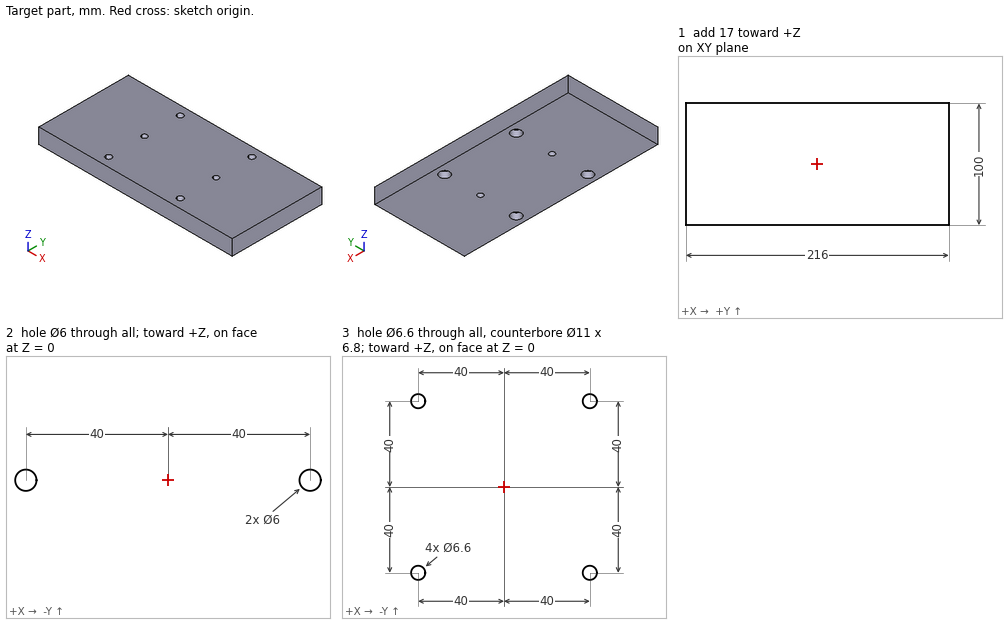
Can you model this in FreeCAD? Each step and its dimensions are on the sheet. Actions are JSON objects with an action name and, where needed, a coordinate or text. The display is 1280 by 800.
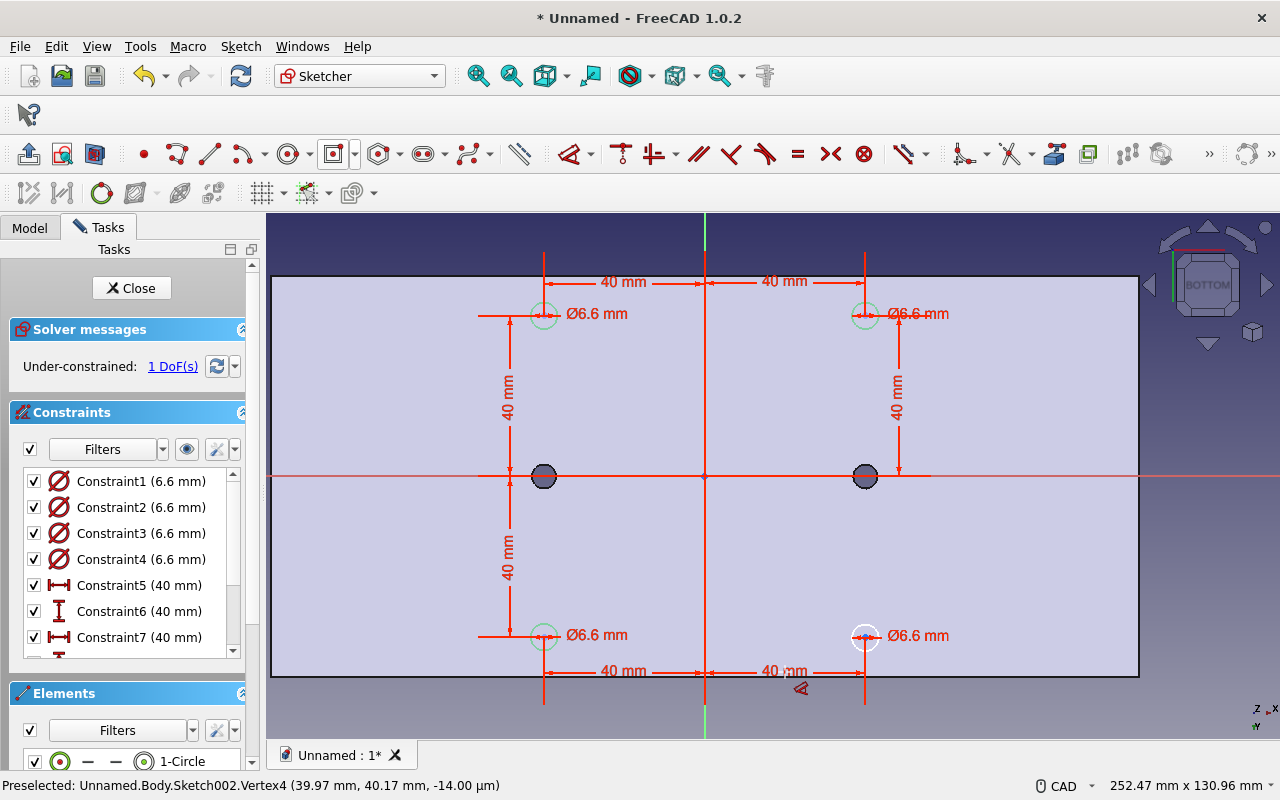
{"action": "left_click", "coordinate": [865, 638]}
{"action": "left_click", "coordinate": [899, 557]}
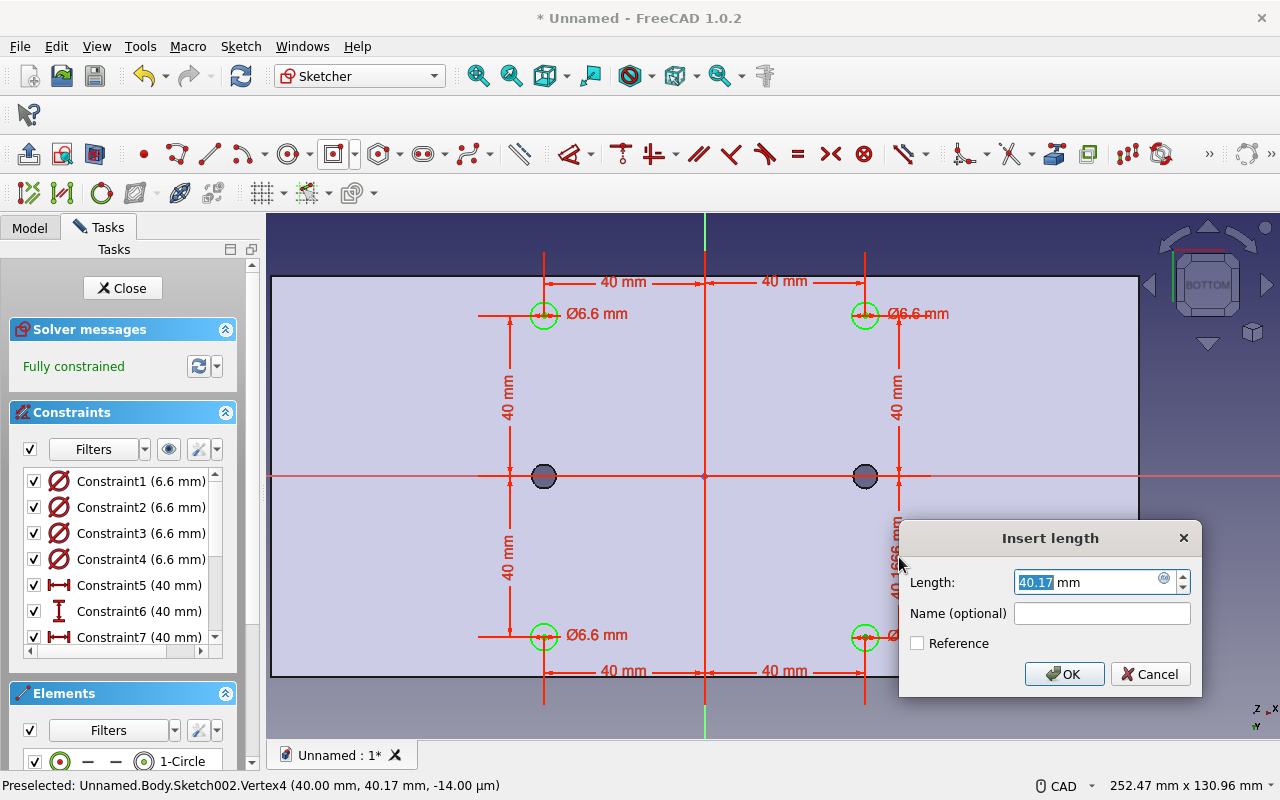
{"action": "type", "text": "40"}
{"action": "key", "text": "Return"}
{"action": "key", "text": "Escape"}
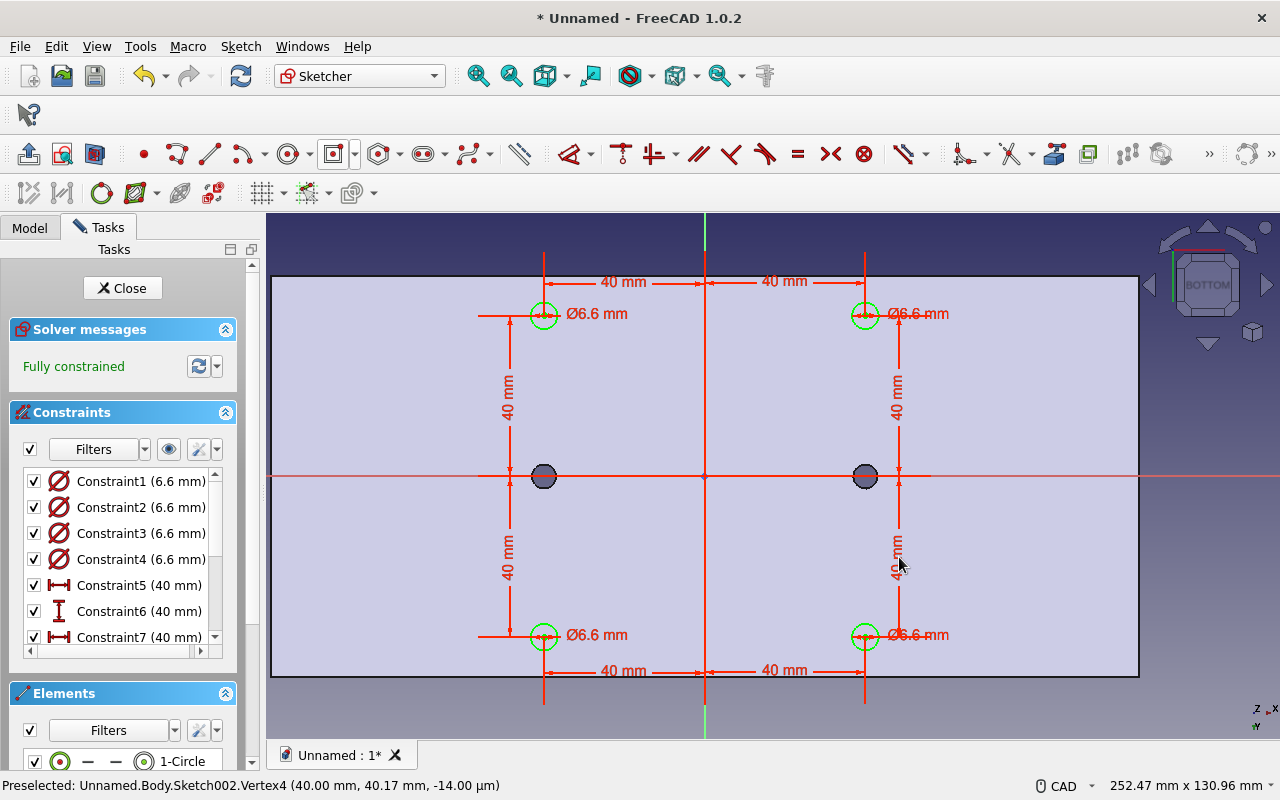
{"action": "left_click", "coordinate": [123, 288]}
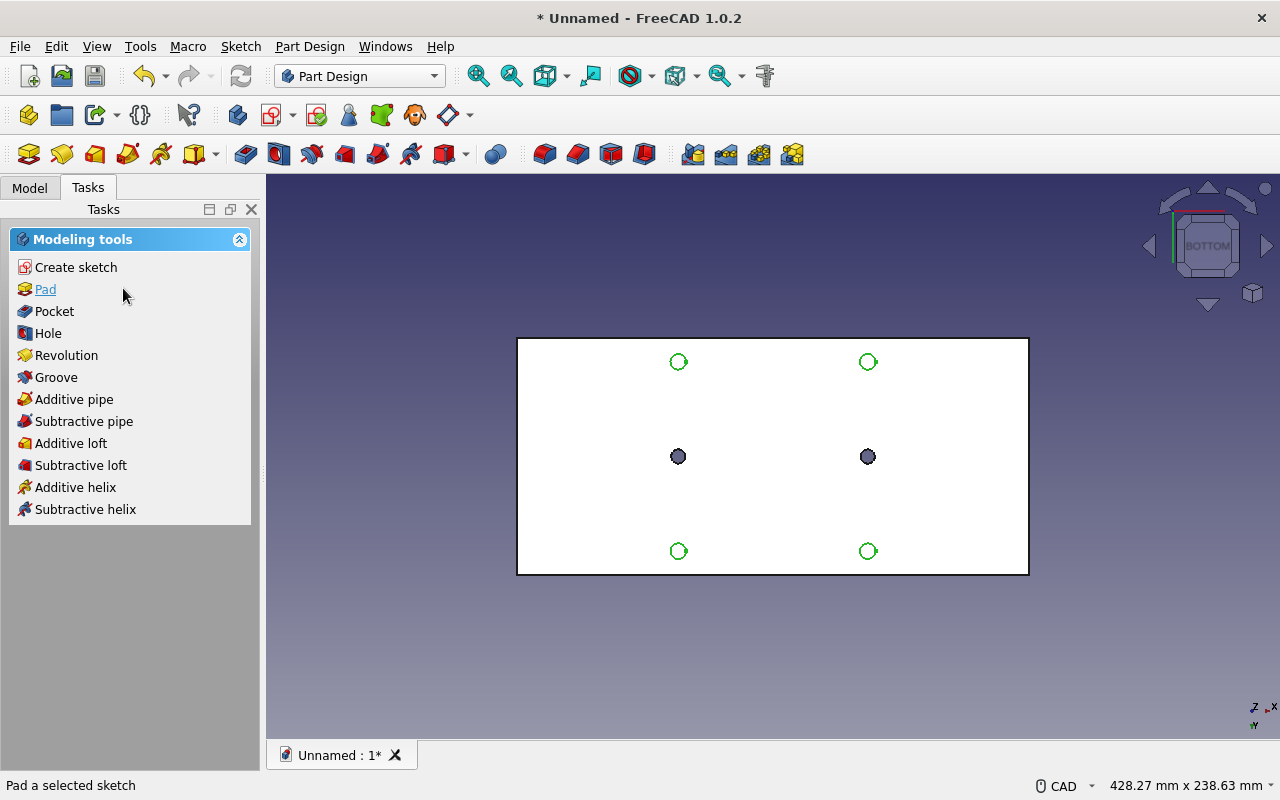
{"action": "left_click", "coordinate": [279, 154]}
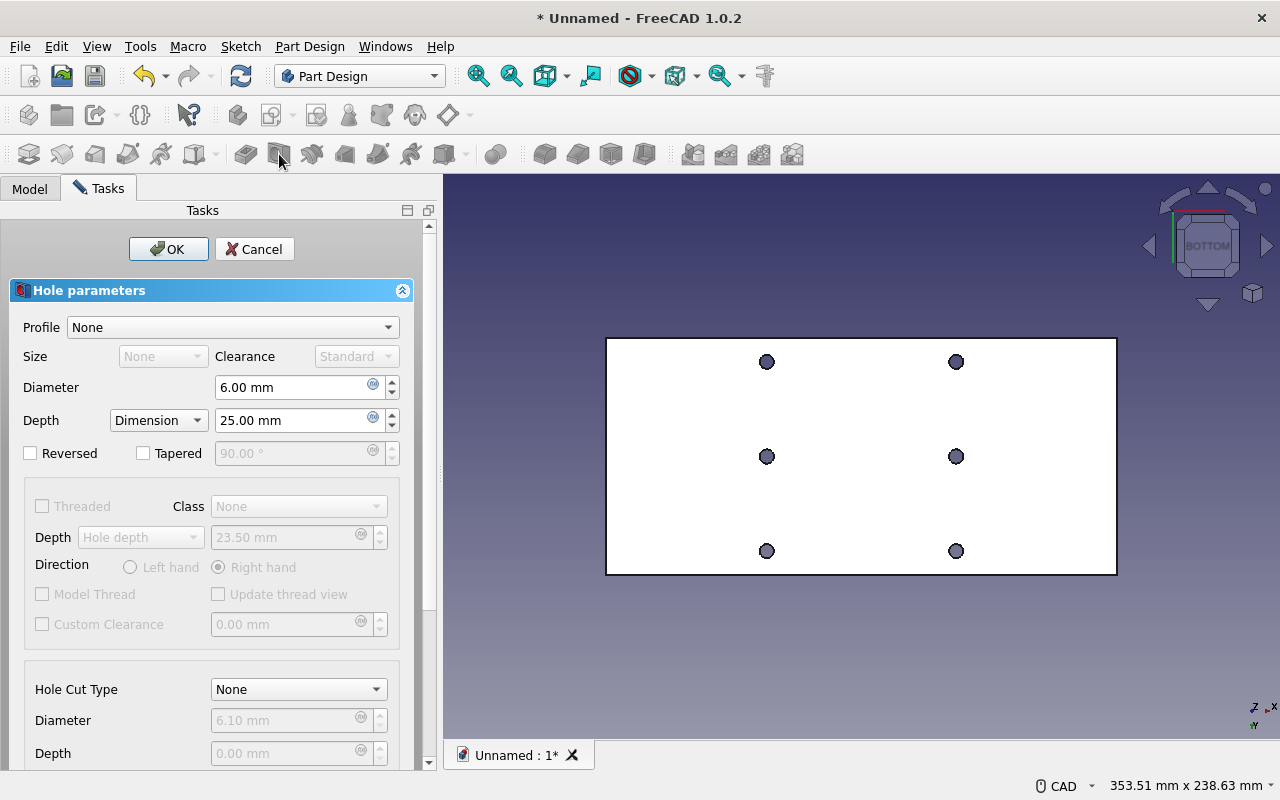
{"action": "triple_click", "coordinate": [300, 388]}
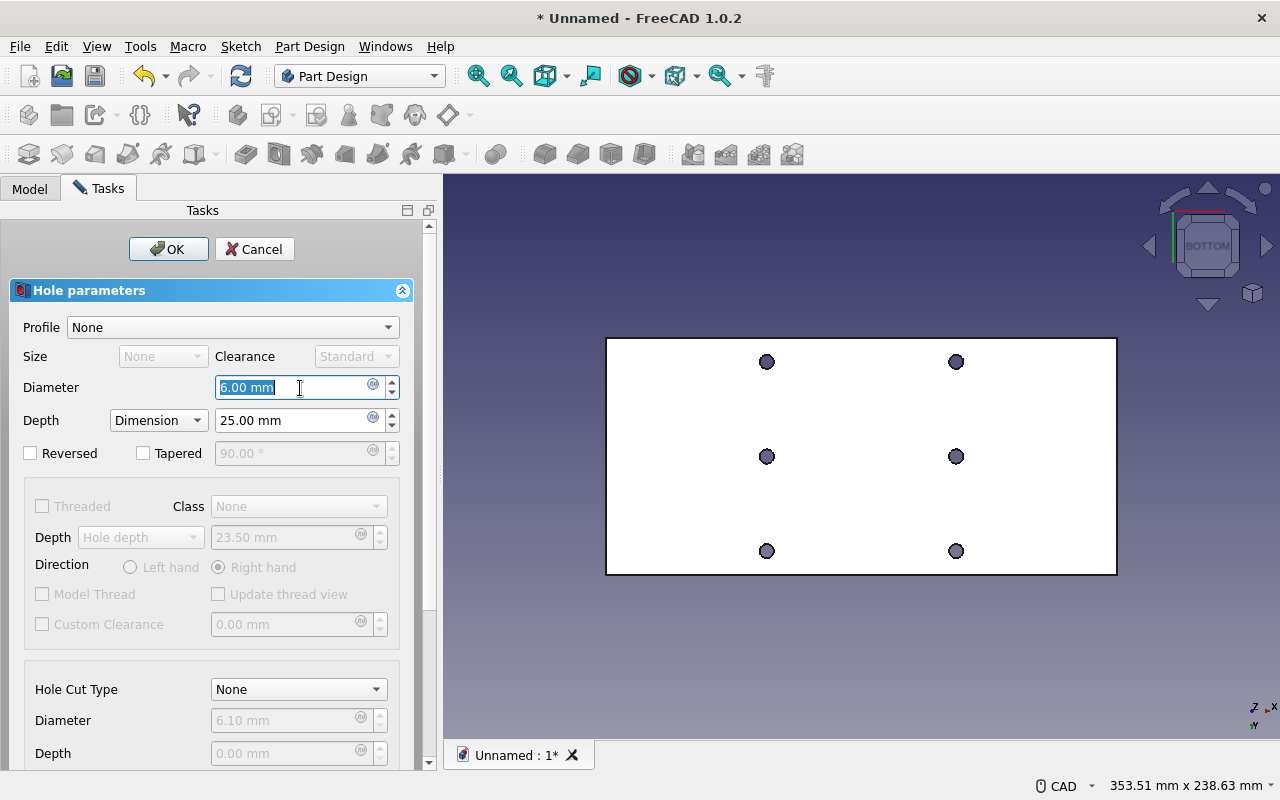
{"action": "type", "text": "6.6"}
{"action": "key", "text": "Tab"}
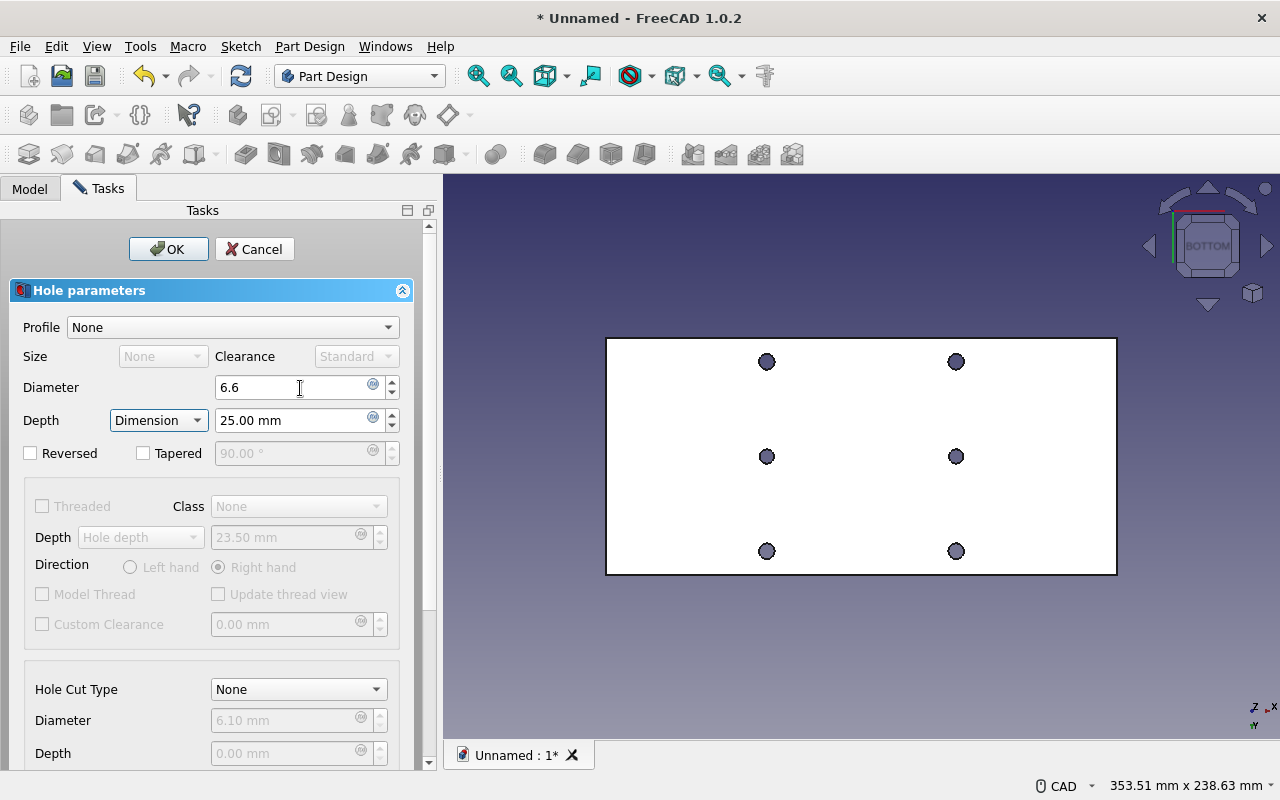
{"action": "left_click", "coordinate": [160, 420]}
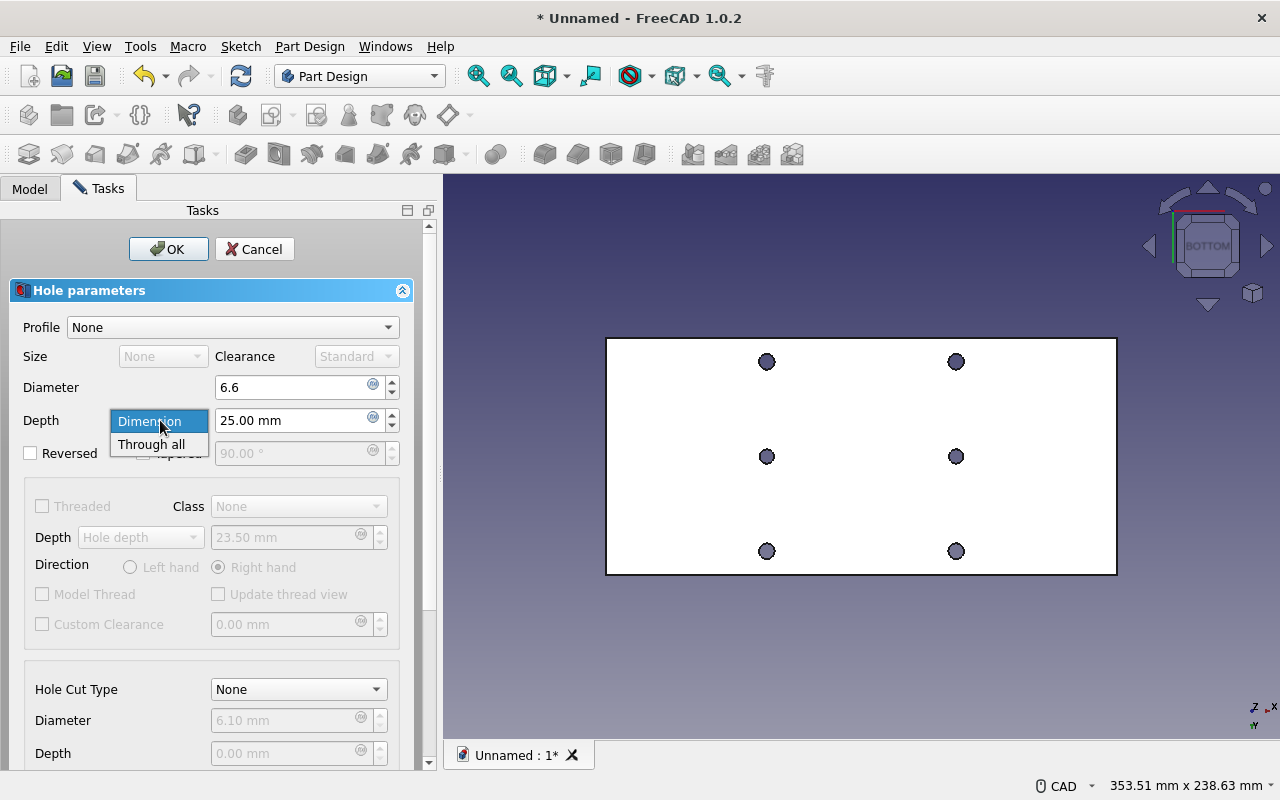
{"action": "left_click", "coordinate": [158, 444]}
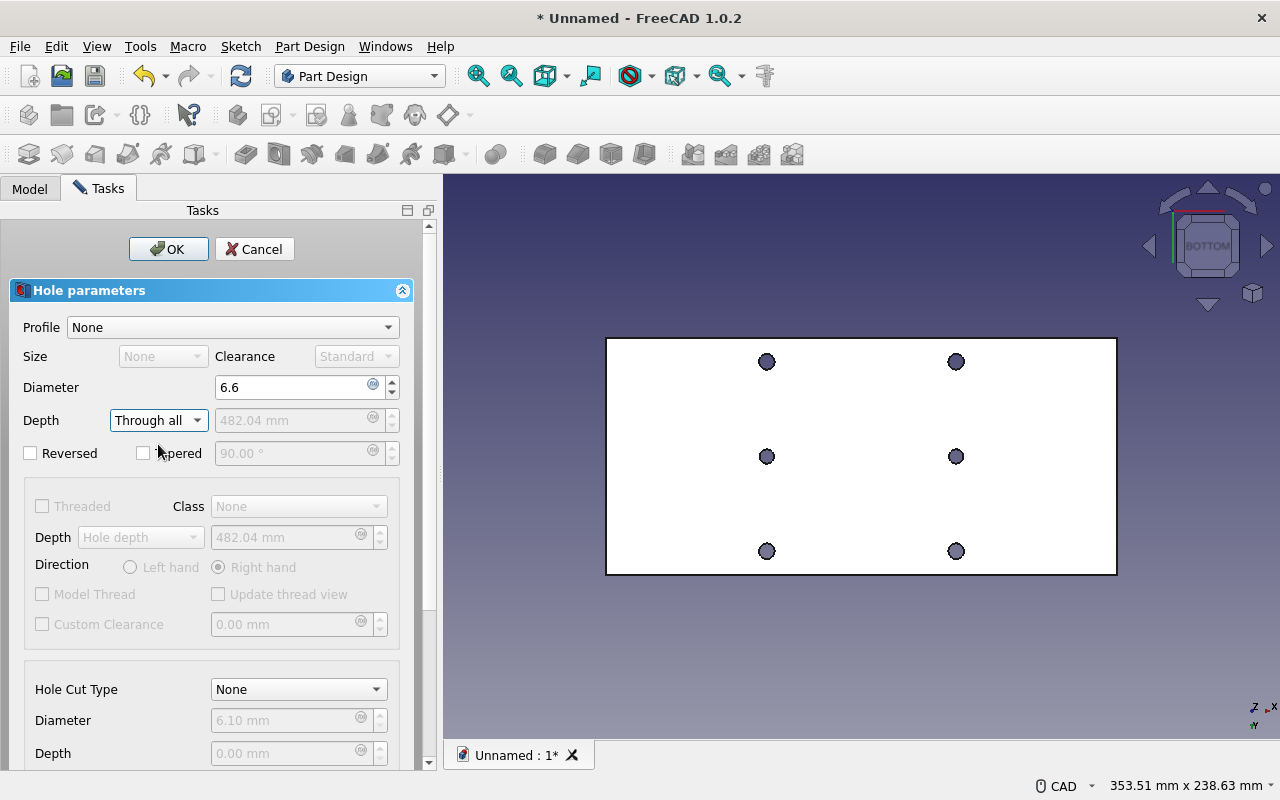
{"action": "left_click", "coordinate": [300, 690]}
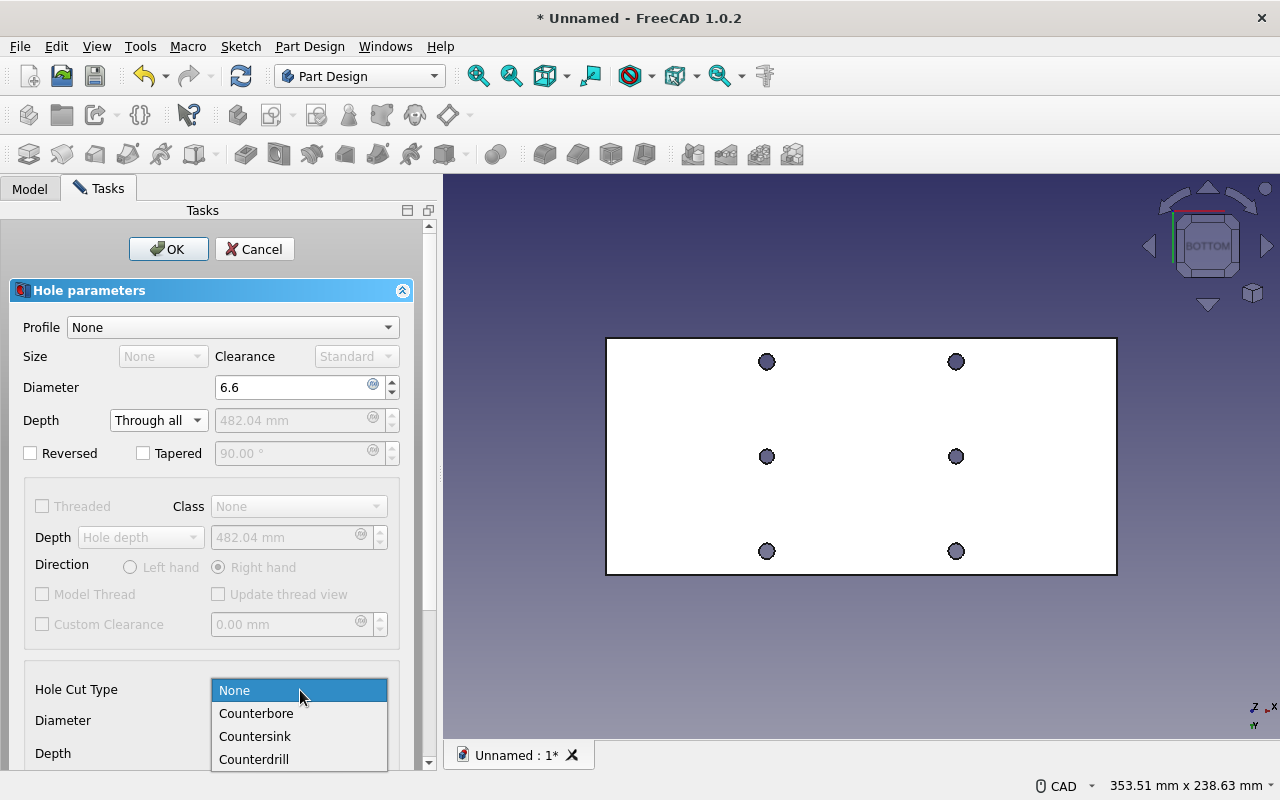
{"action": "left_click", "coordinate": [298, 714]}